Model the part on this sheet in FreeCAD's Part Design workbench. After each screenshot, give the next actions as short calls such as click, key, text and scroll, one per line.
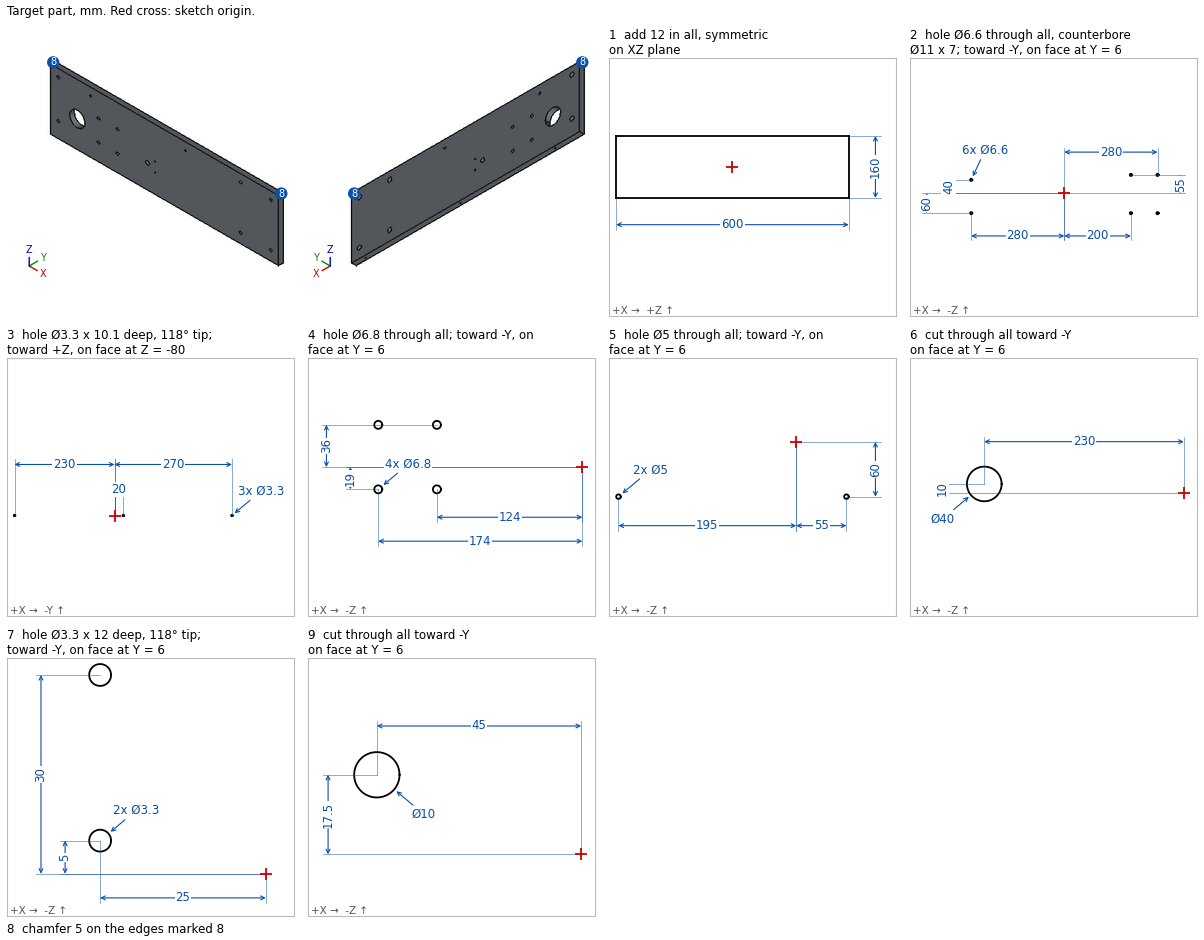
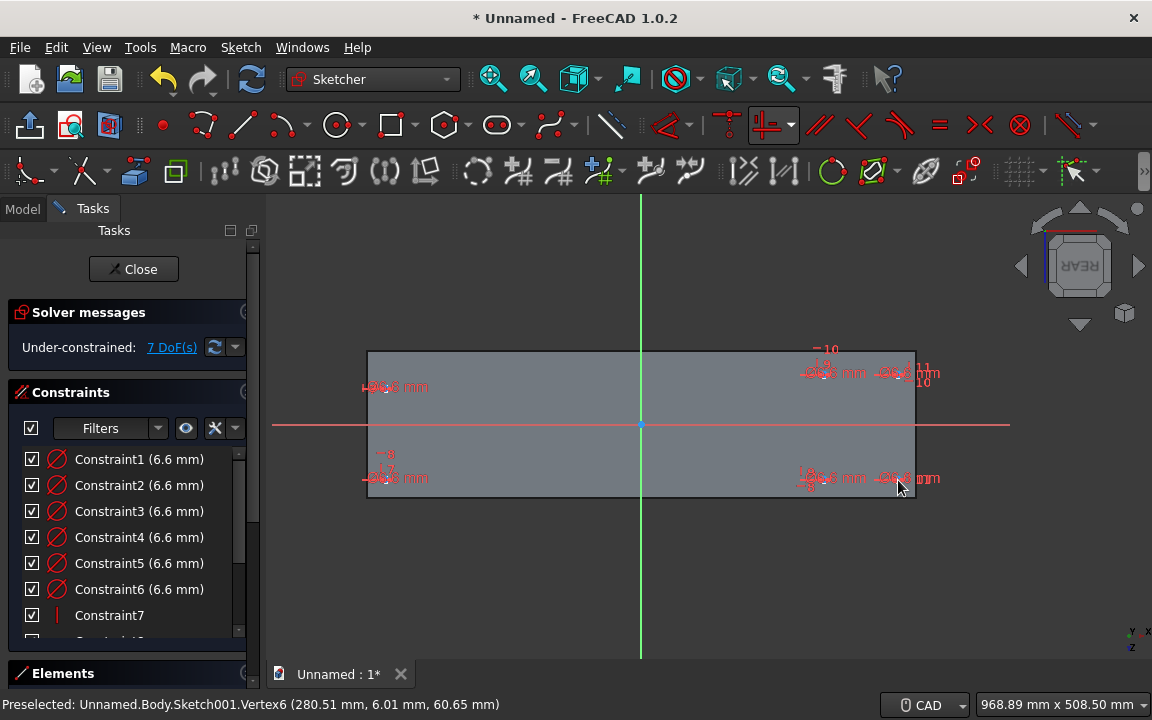
click(824, 480)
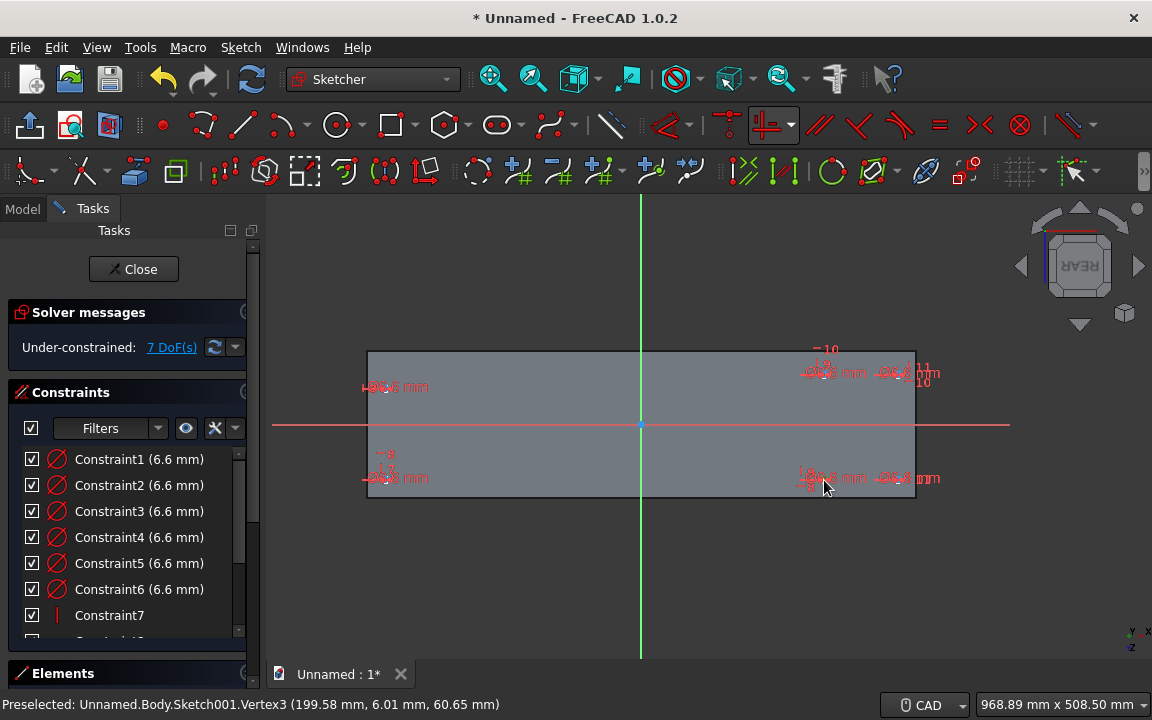
click(898, 480)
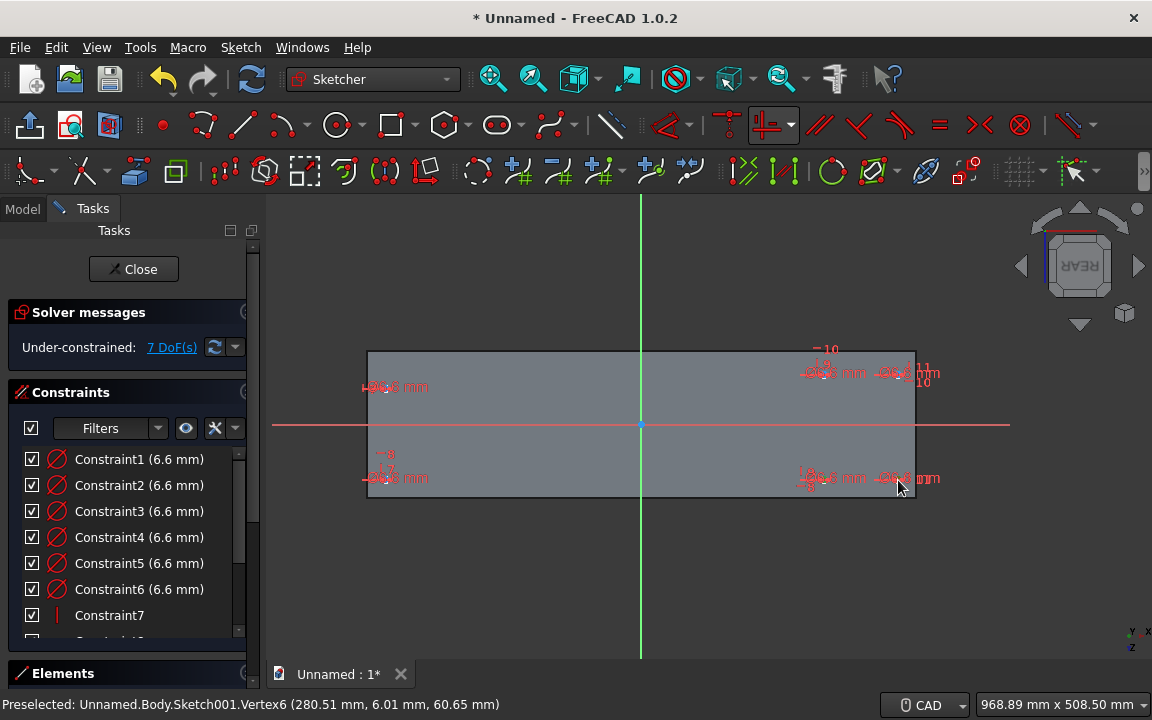
click(794, 126)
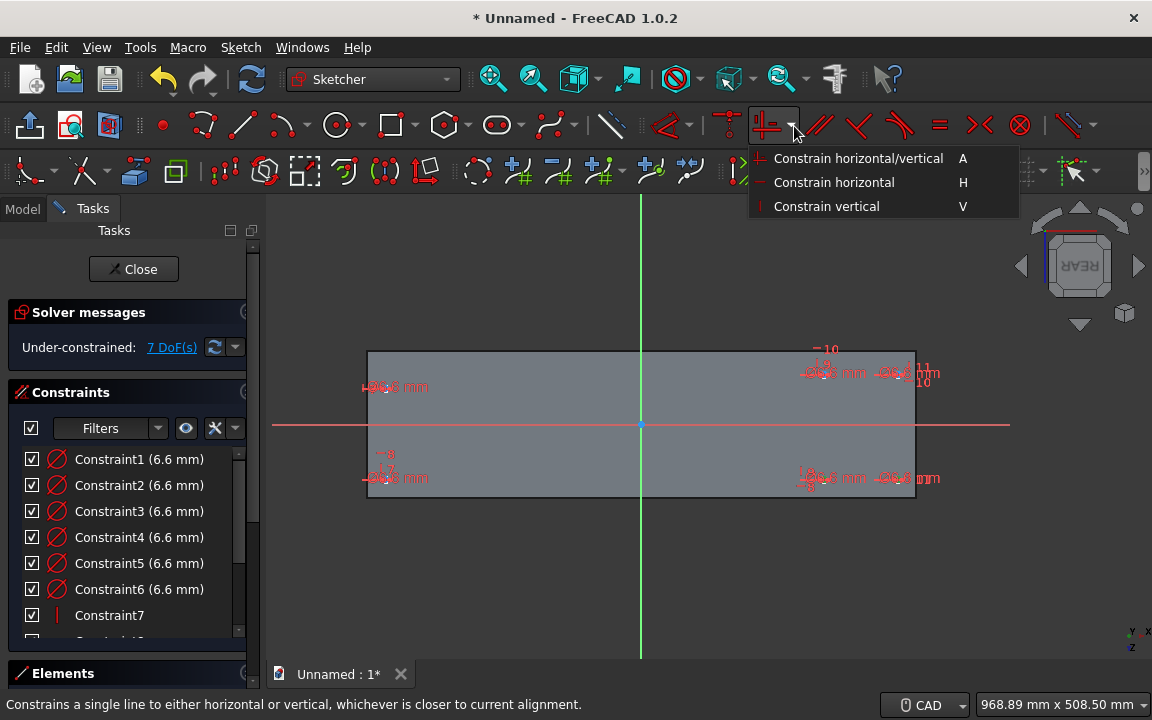
click(884, 182)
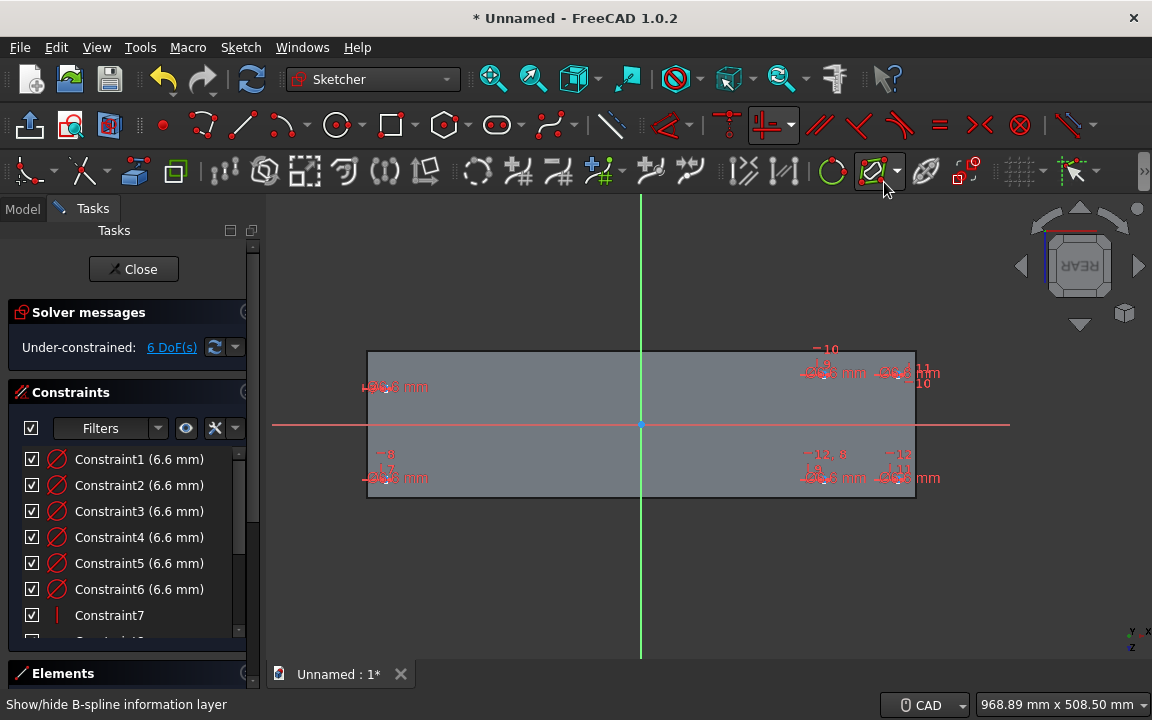
click(386, 480)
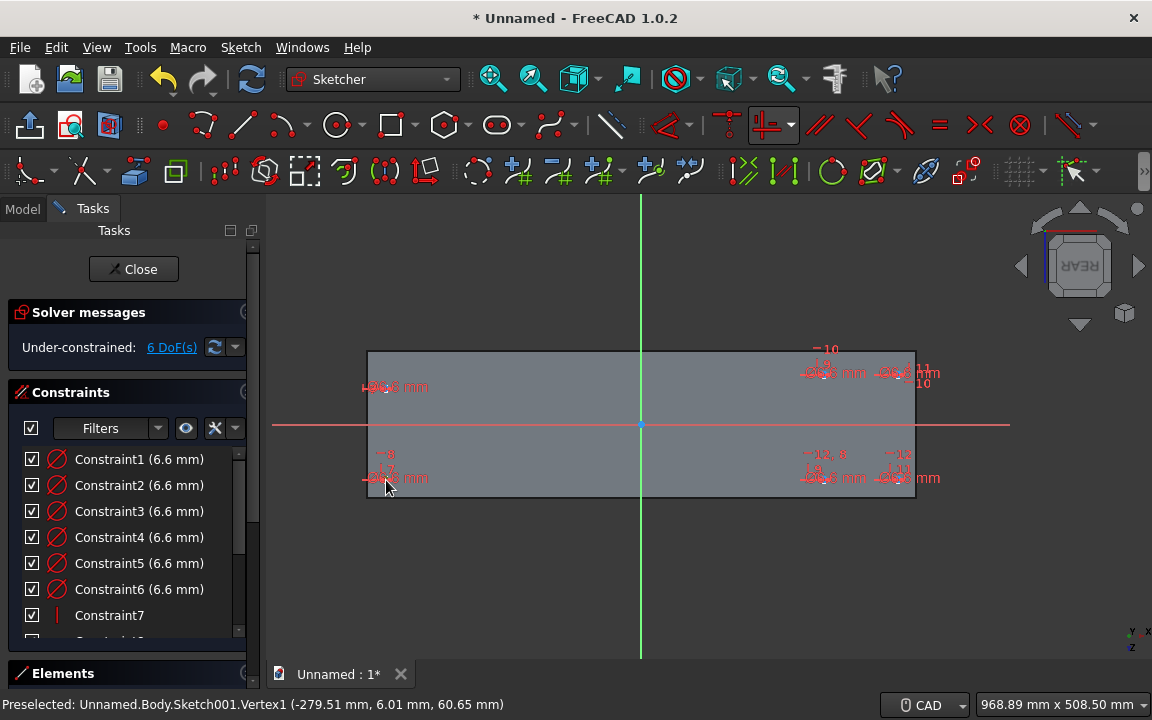
key(i)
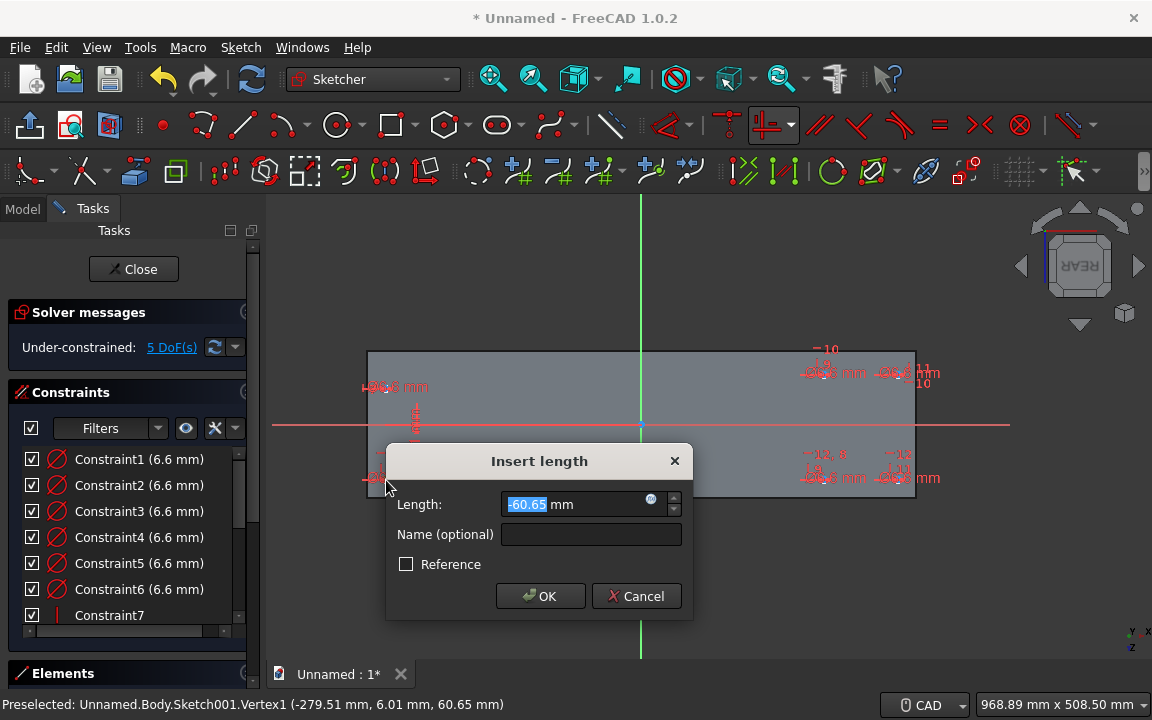
text(-60)
key(Return)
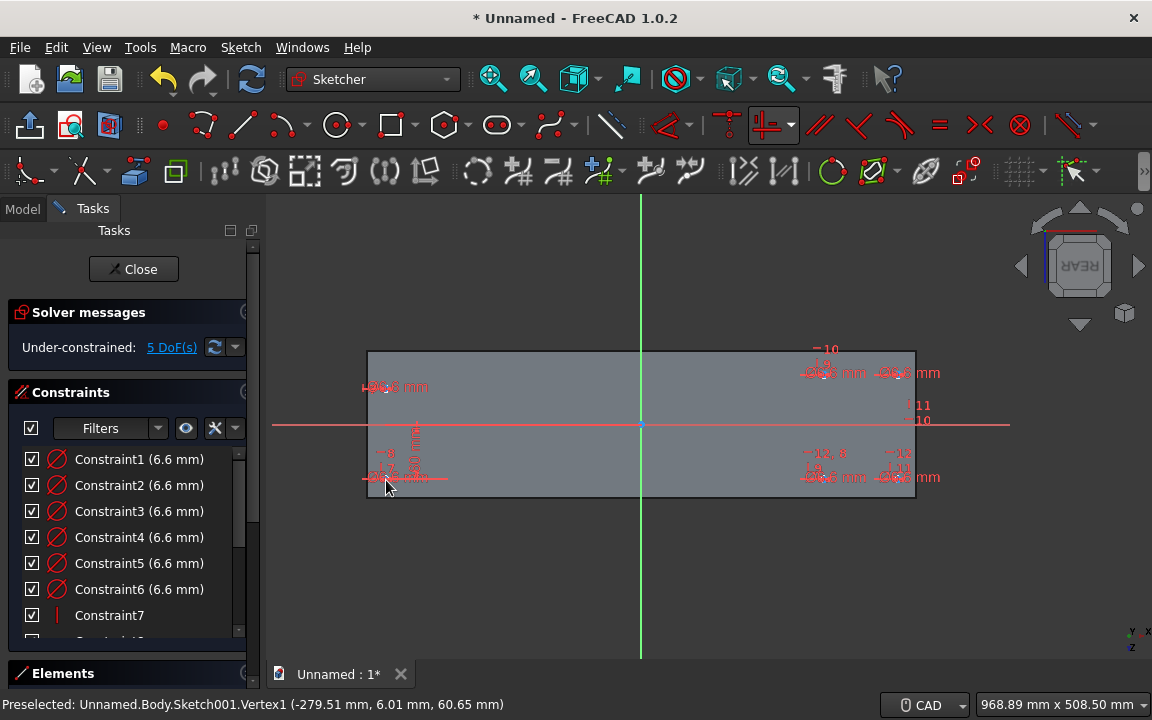
click(386, 389)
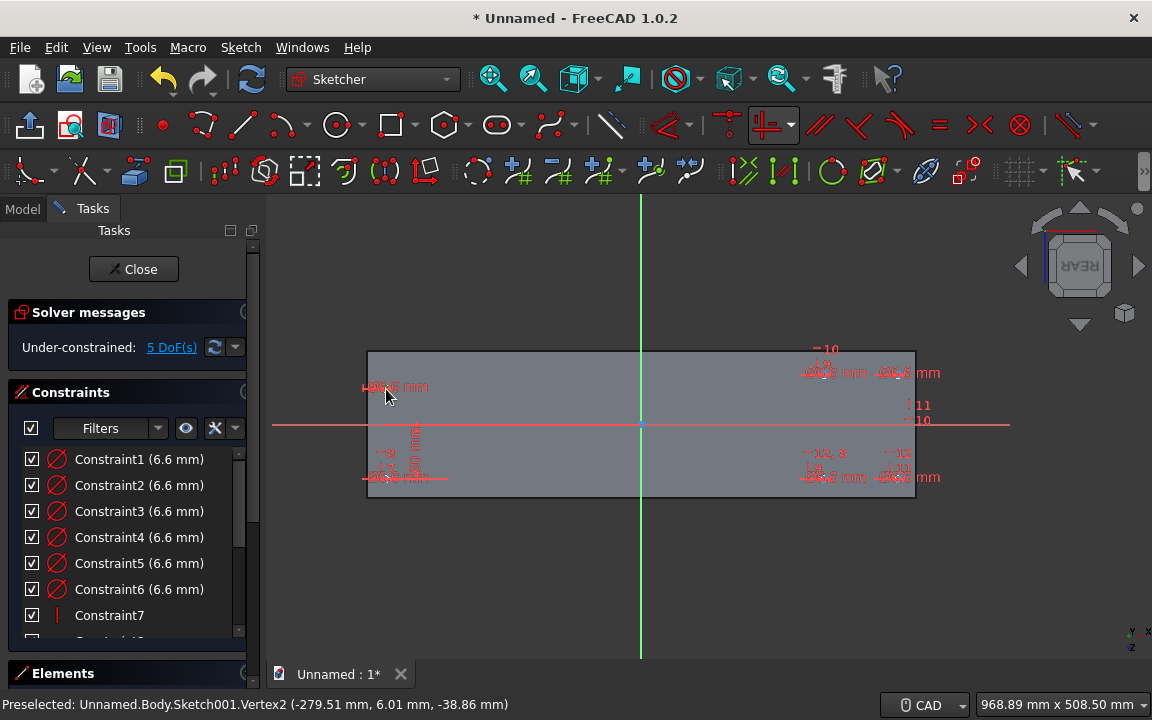
key(i)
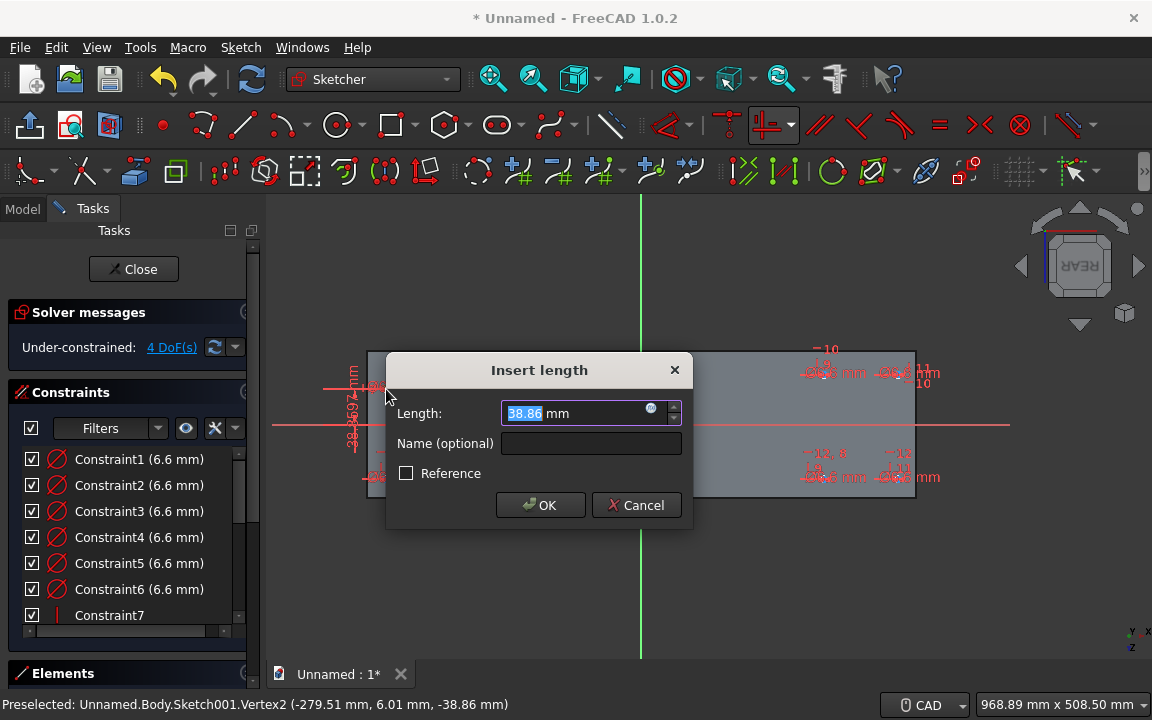
text(40)
key(Return)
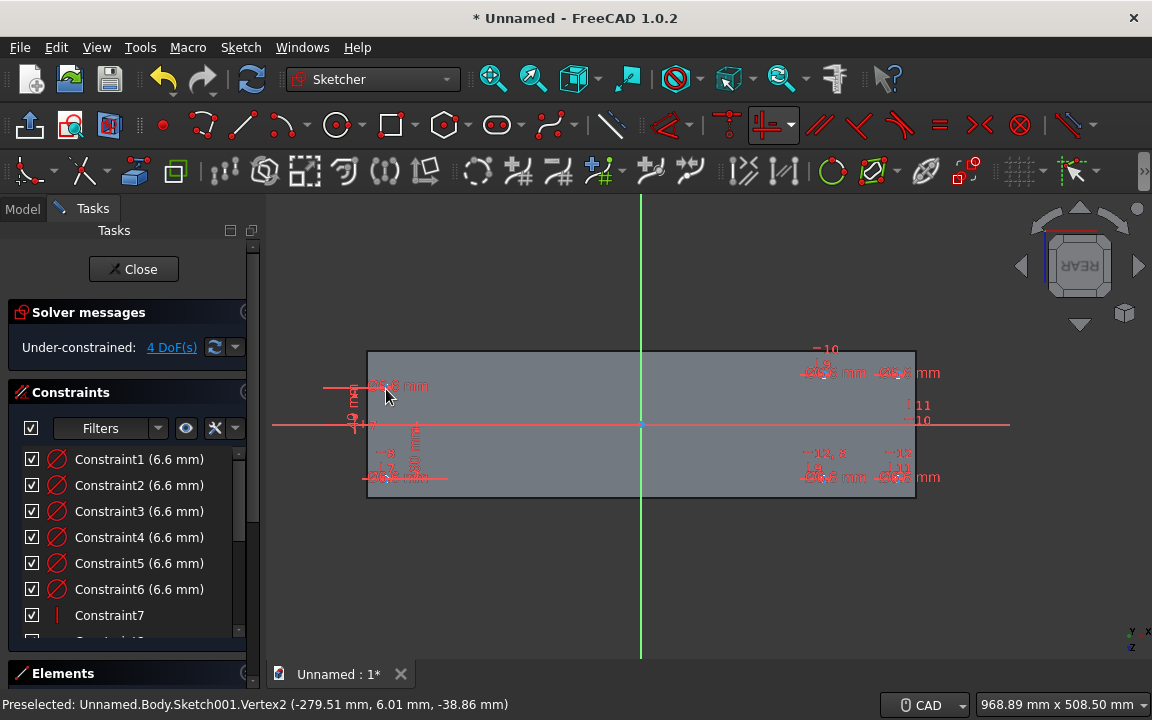
click(824, 375)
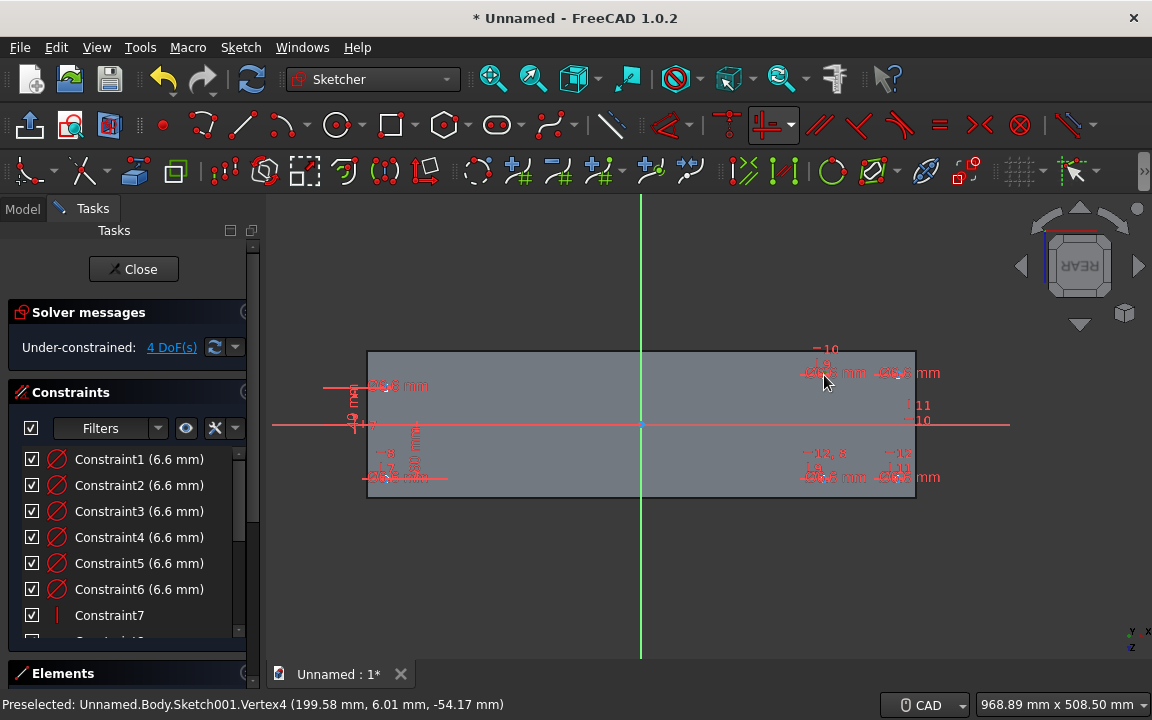
click(692, 126)